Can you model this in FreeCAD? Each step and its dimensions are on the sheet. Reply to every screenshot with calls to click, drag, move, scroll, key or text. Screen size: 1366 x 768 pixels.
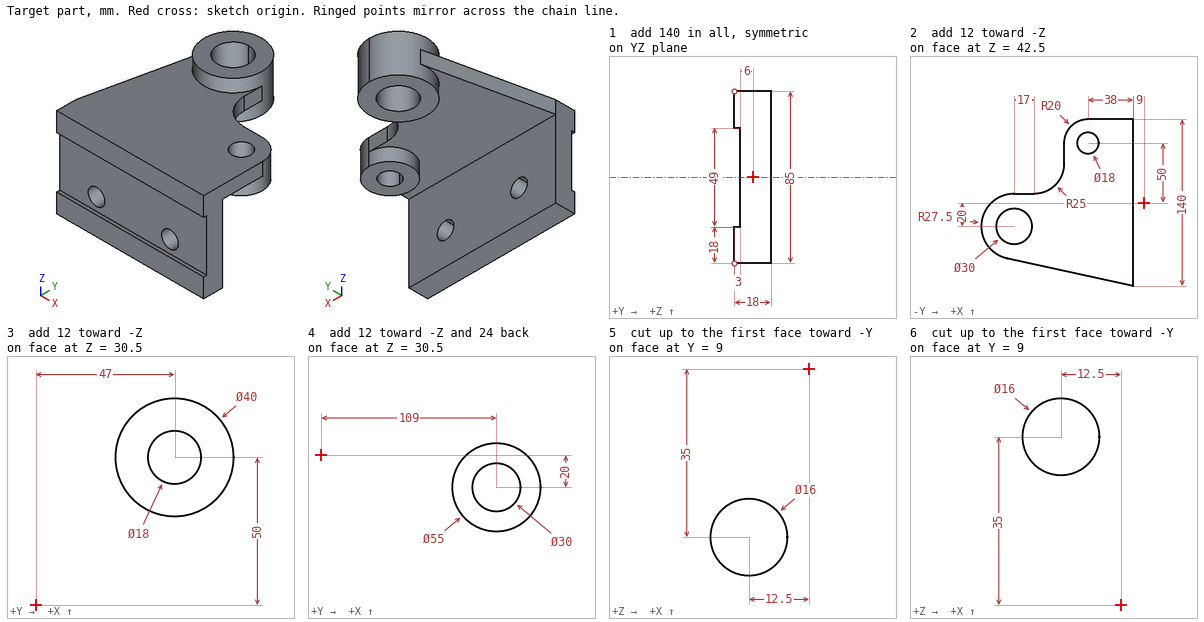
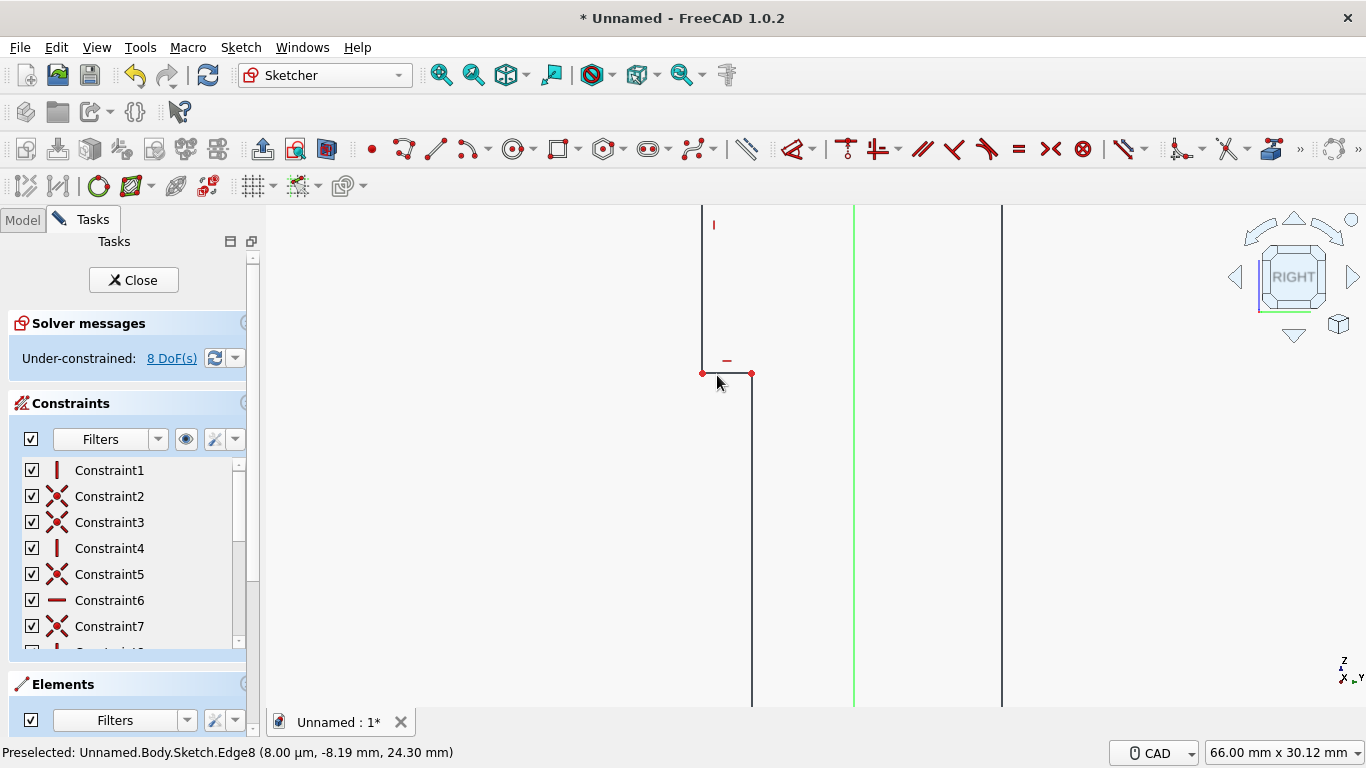
scroll(721, 374, down, 8)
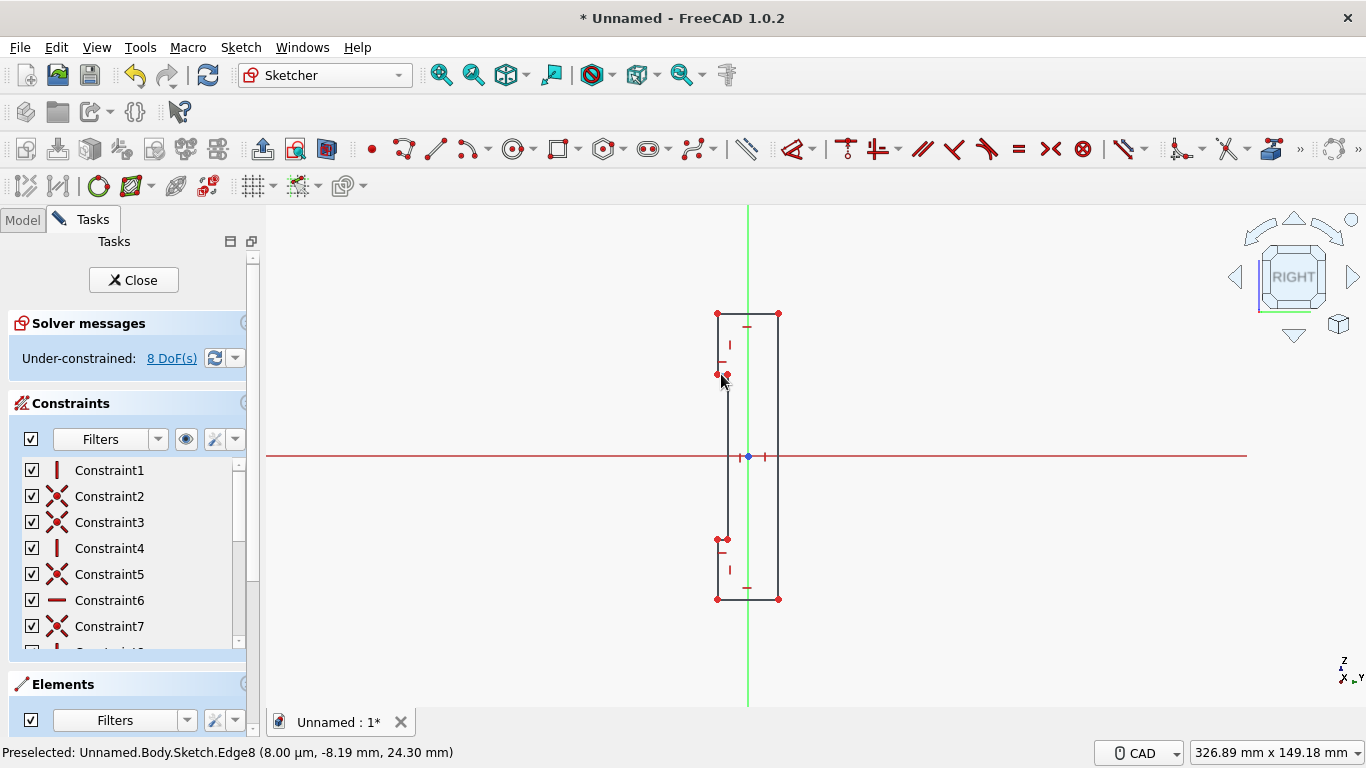
click(718, 600)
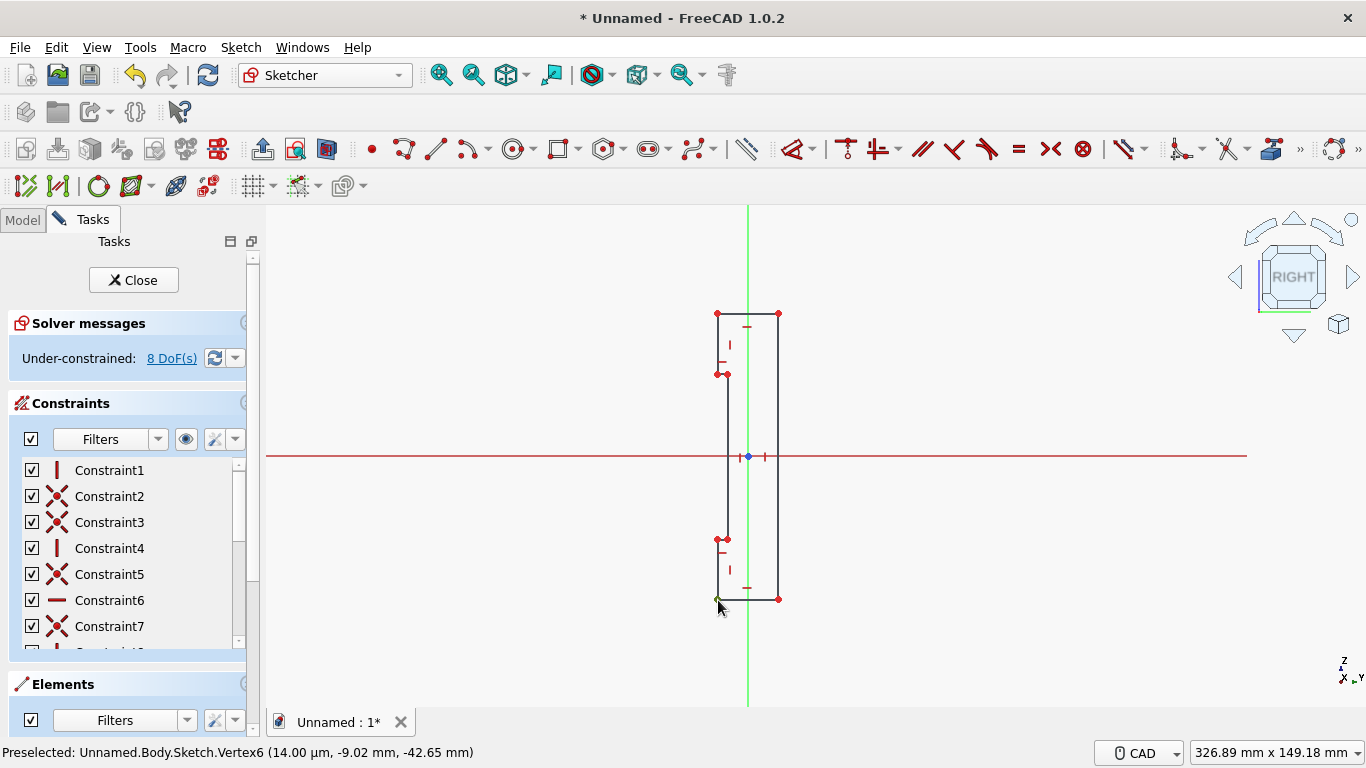
click(718, 314)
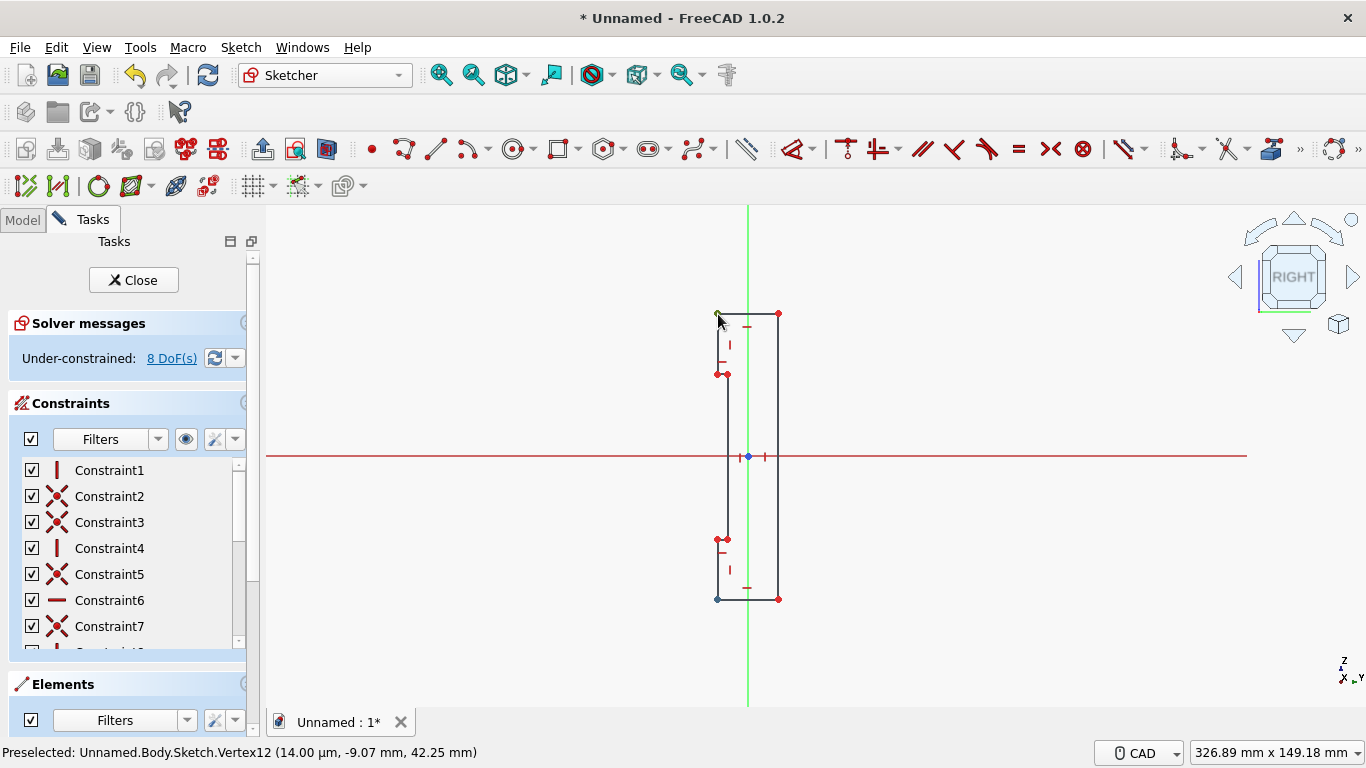
click(359, 456)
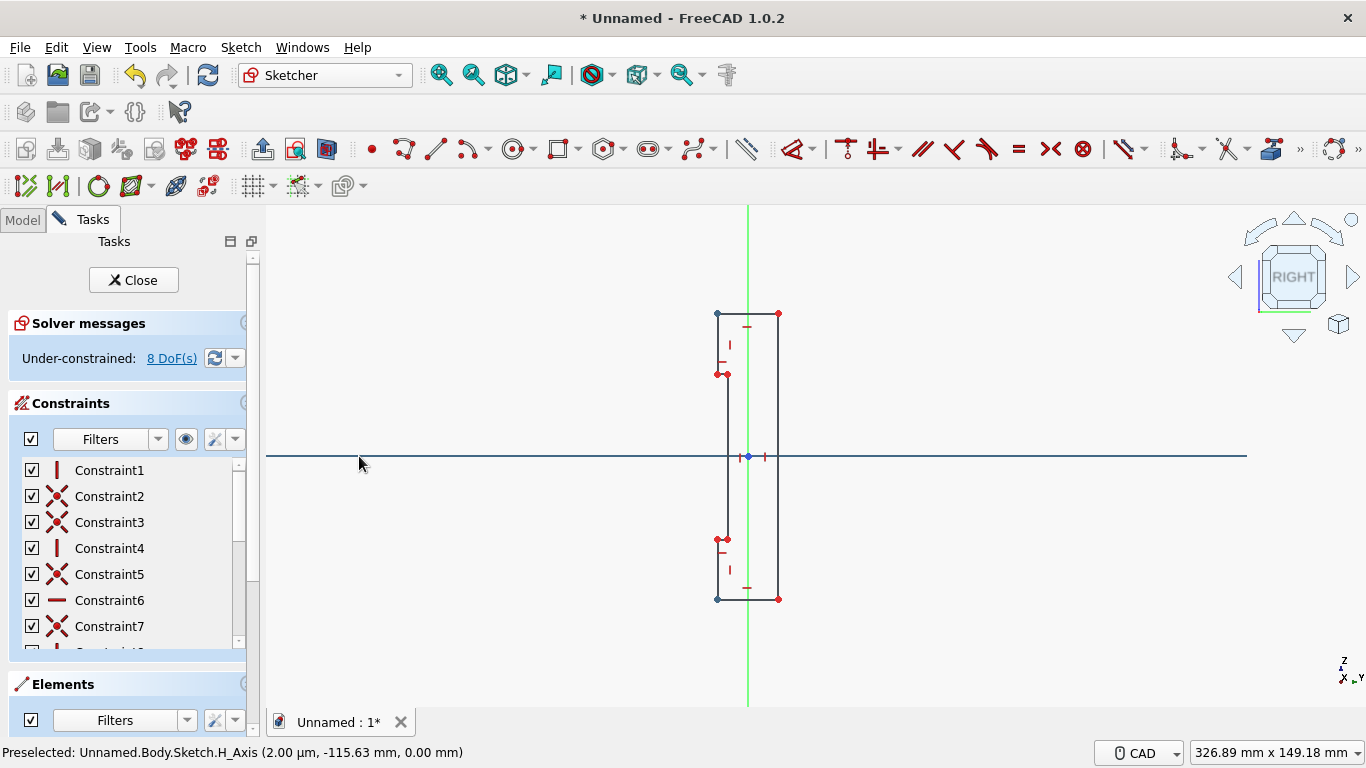
click(1052, 150)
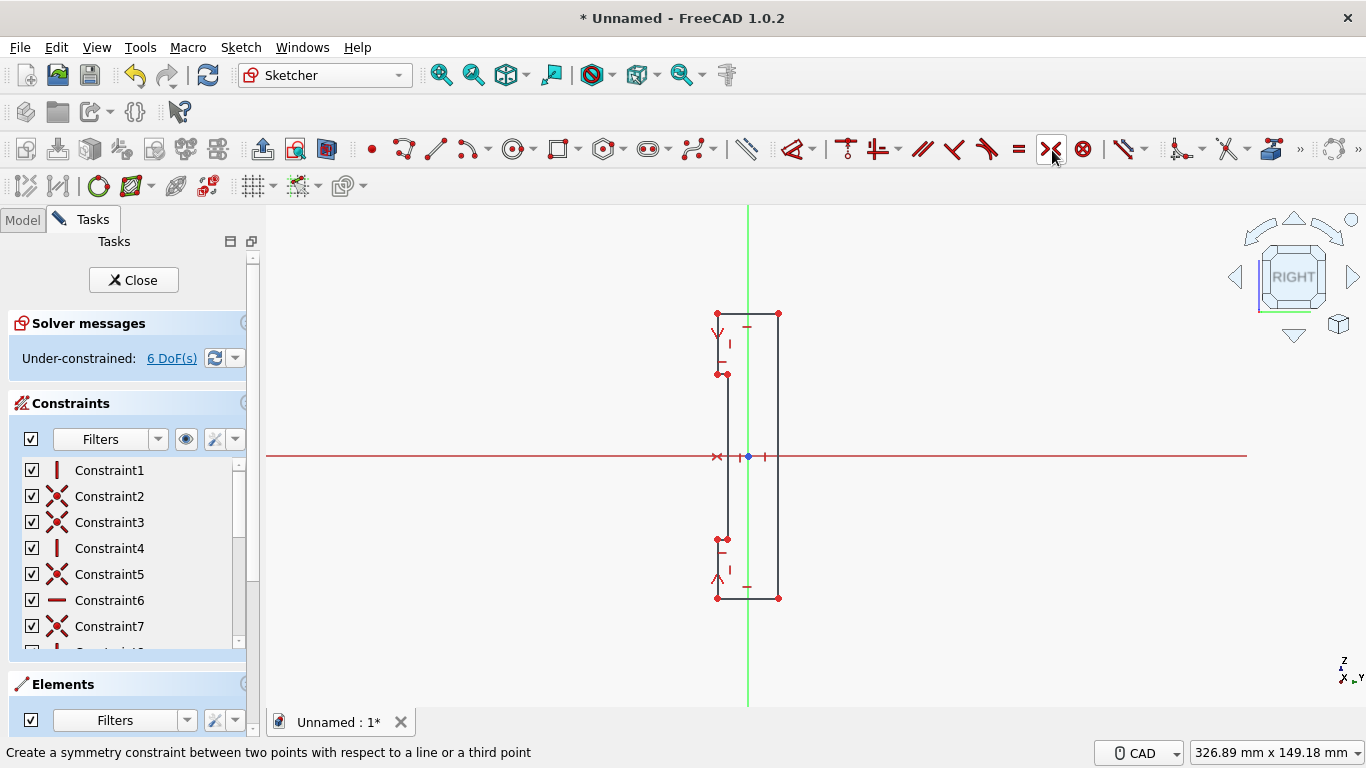
scroll(723, 540, up, 7)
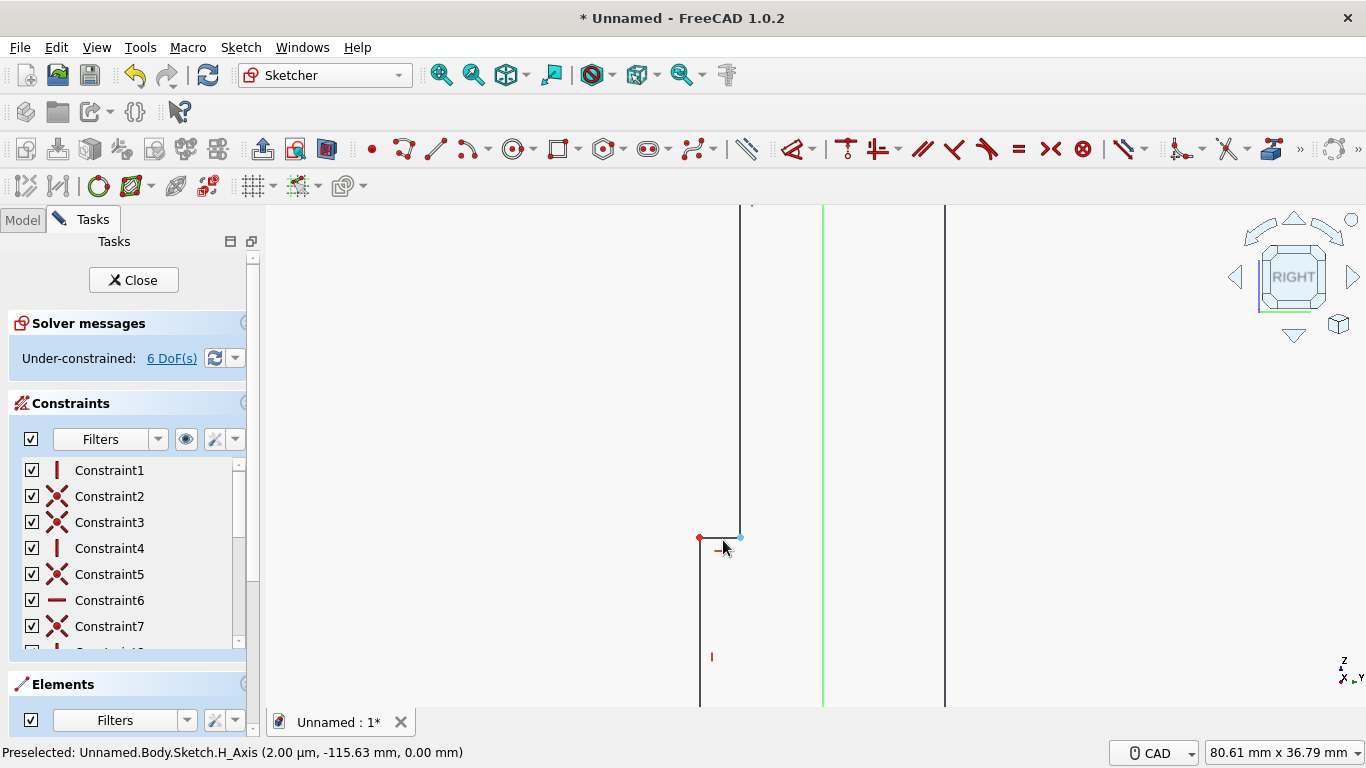
click(720, 538)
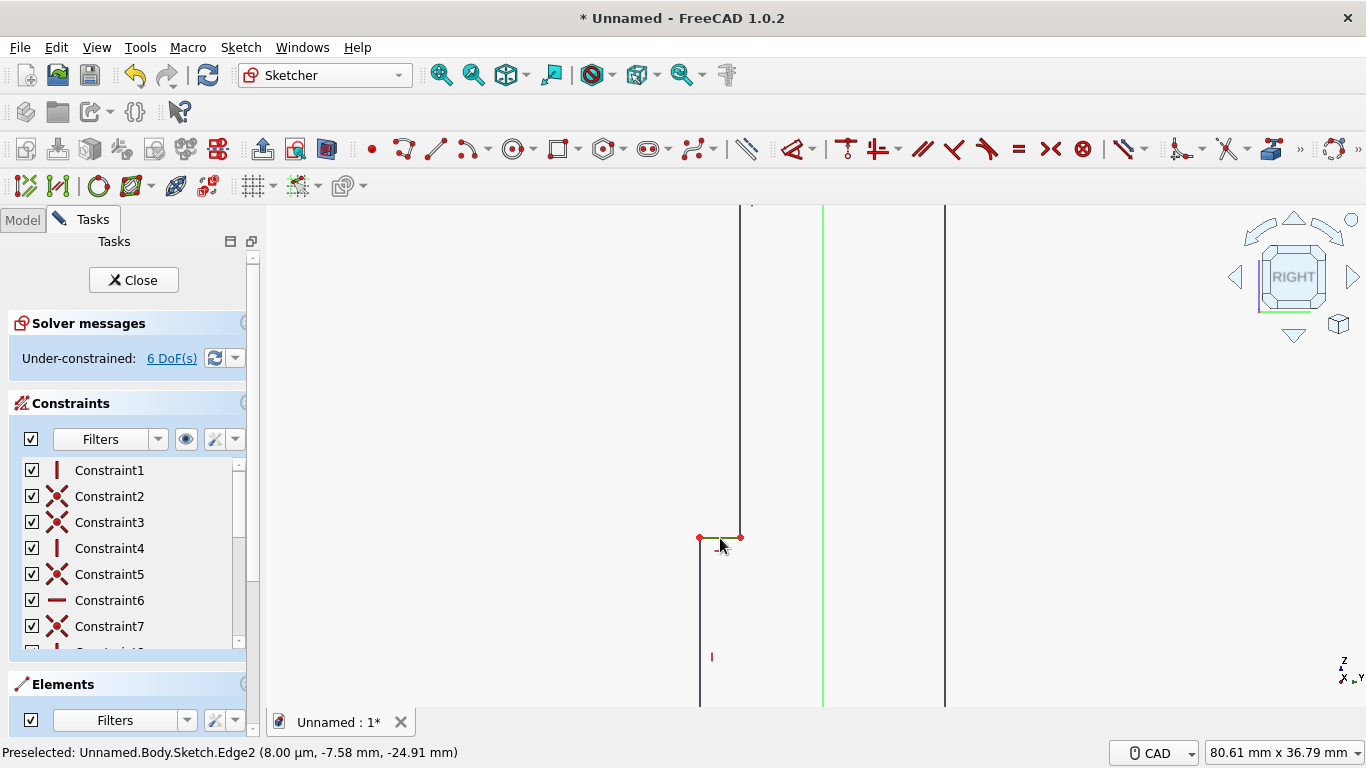
key(l)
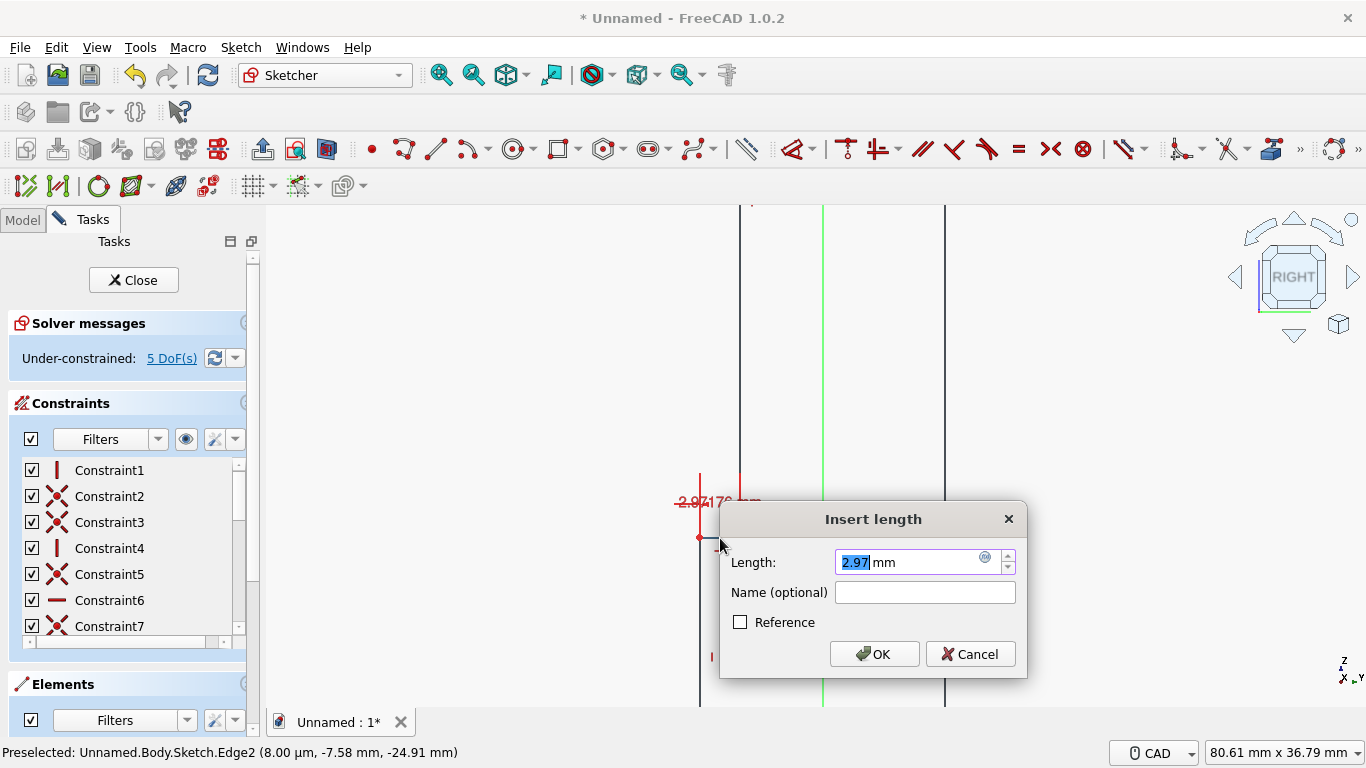
text(3)
key(Return)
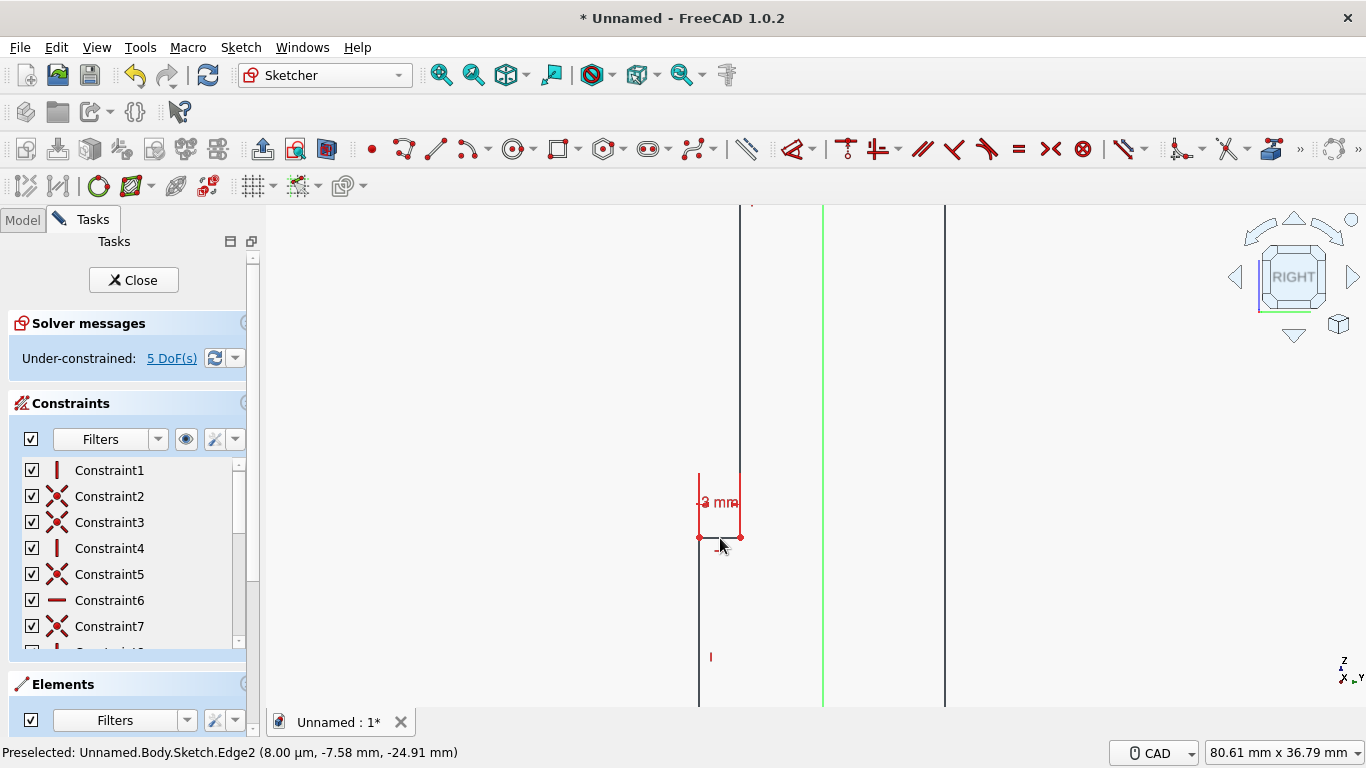
scroll(723, 540, down, 7)